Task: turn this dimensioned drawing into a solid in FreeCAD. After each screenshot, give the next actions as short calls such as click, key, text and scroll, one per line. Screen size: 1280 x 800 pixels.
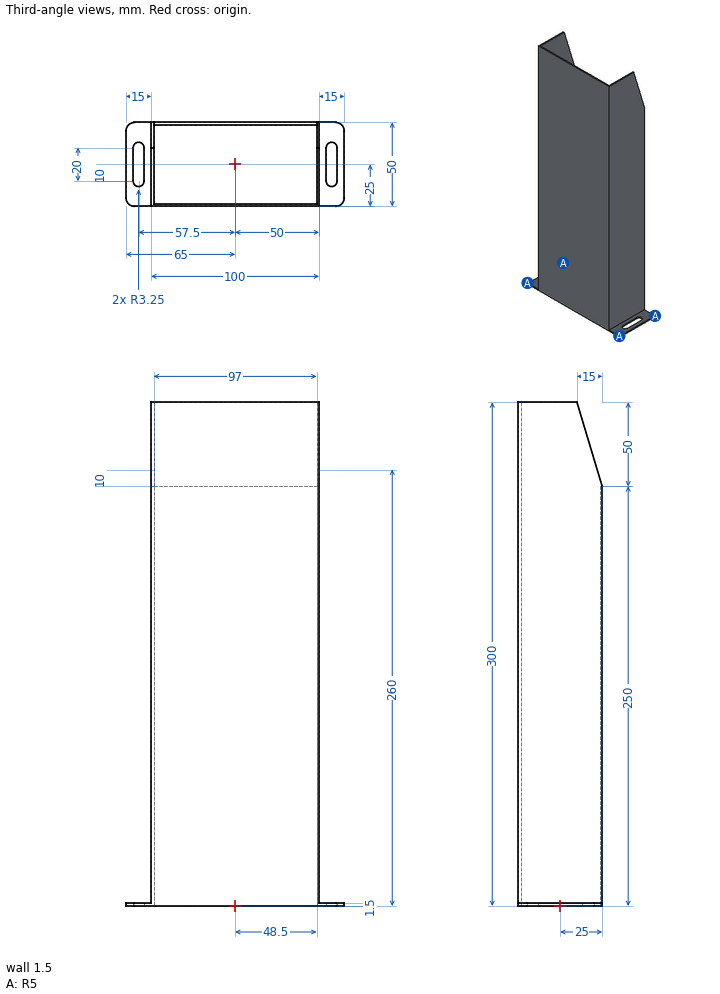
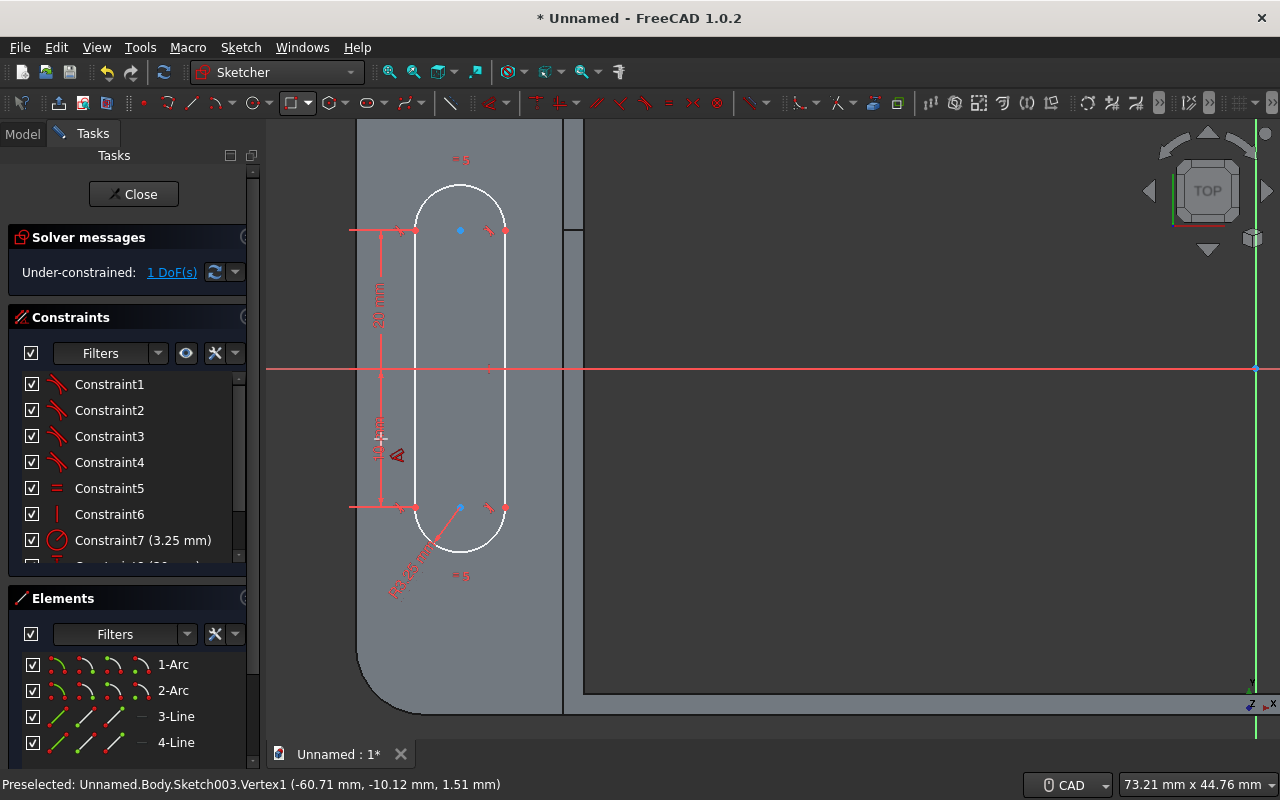
click(460, 507)
click(788, 541)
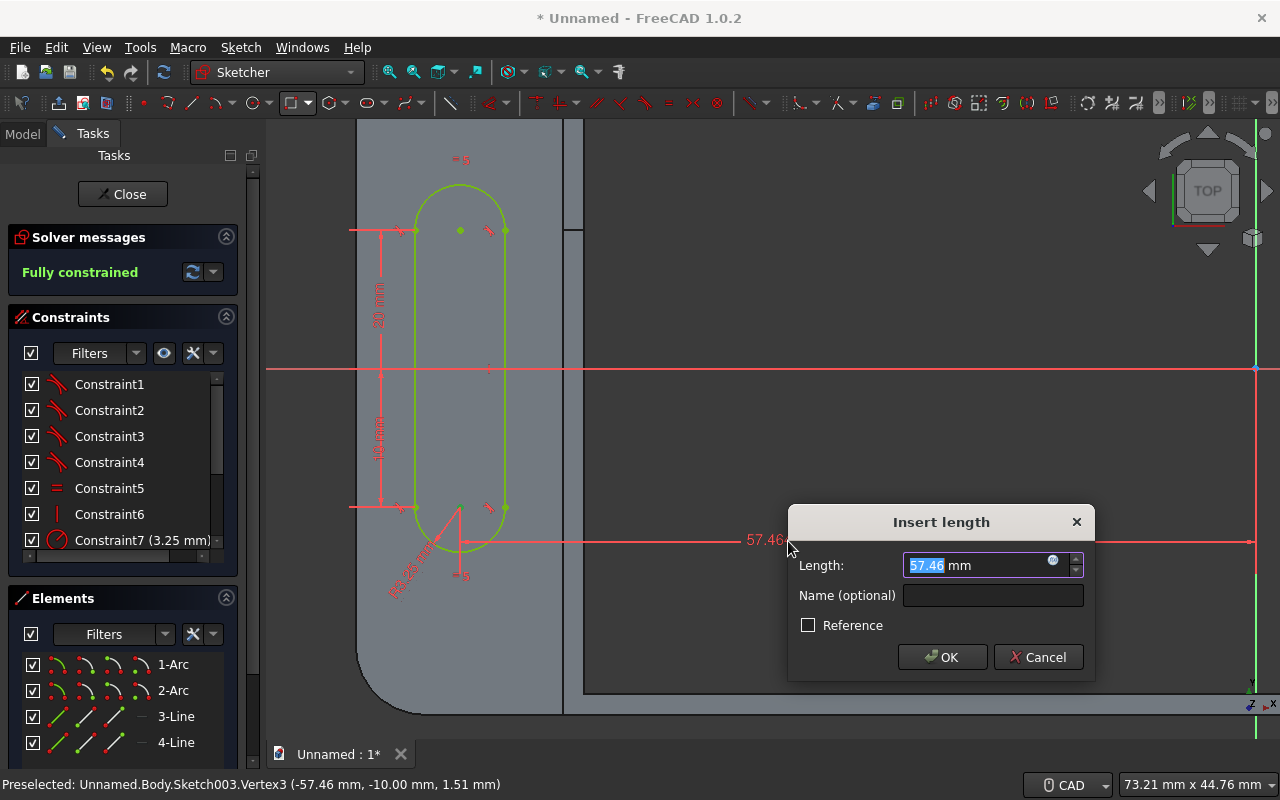
text(57.5)
key(Return)
key(Escape)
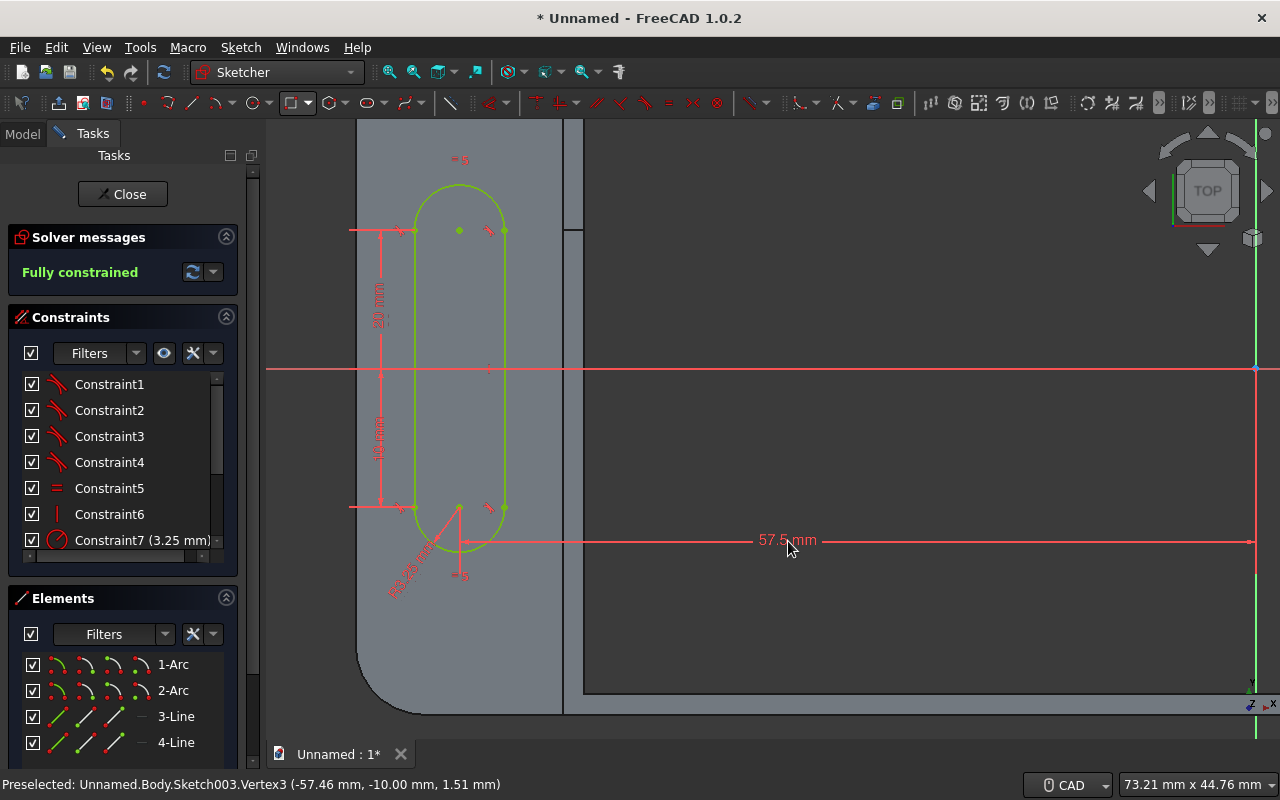
click(123, 194)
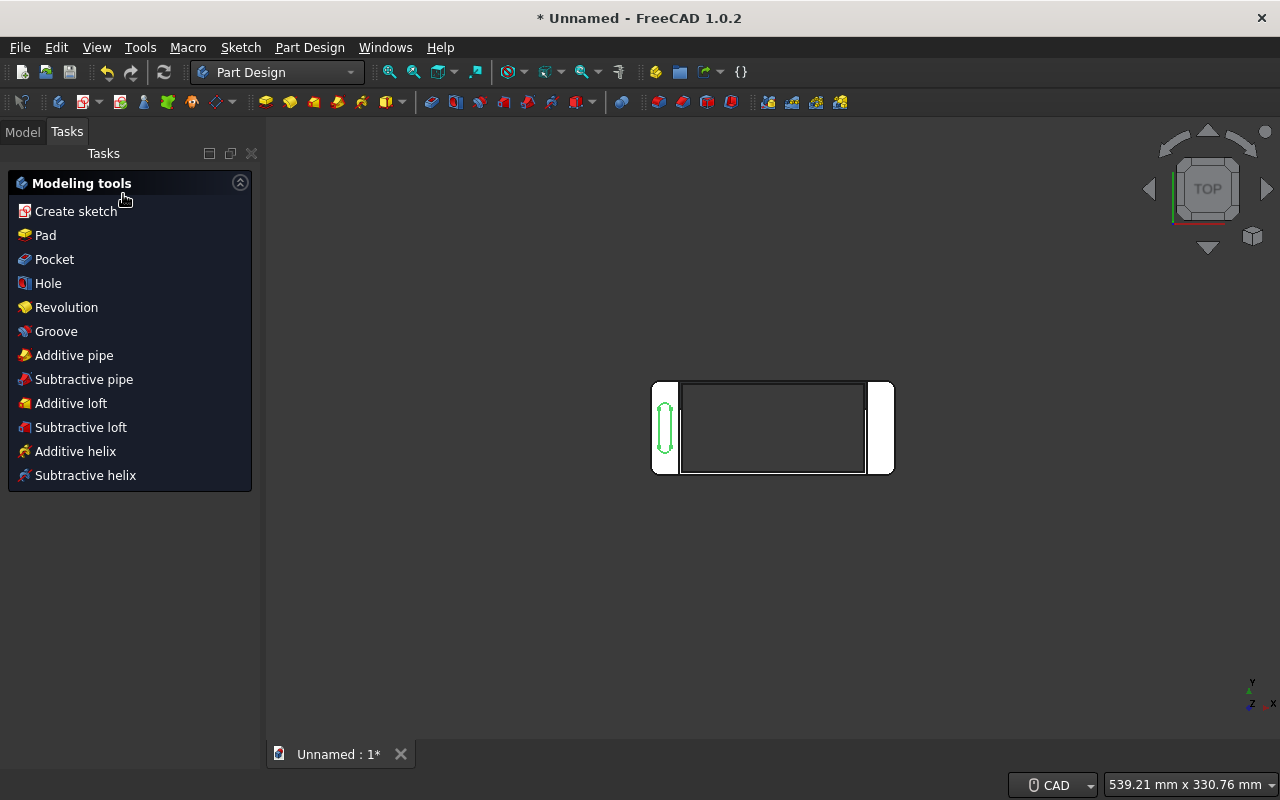
click(432, 102)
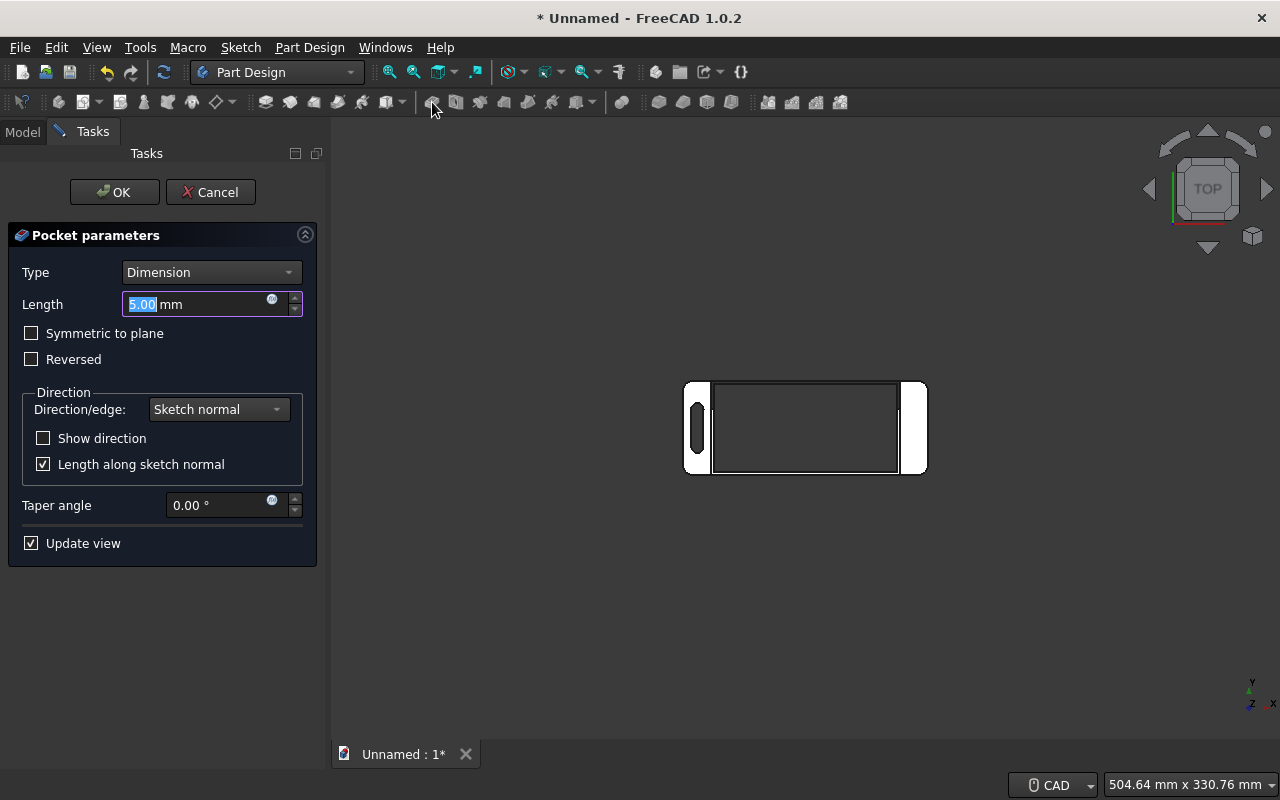
click(212, 272)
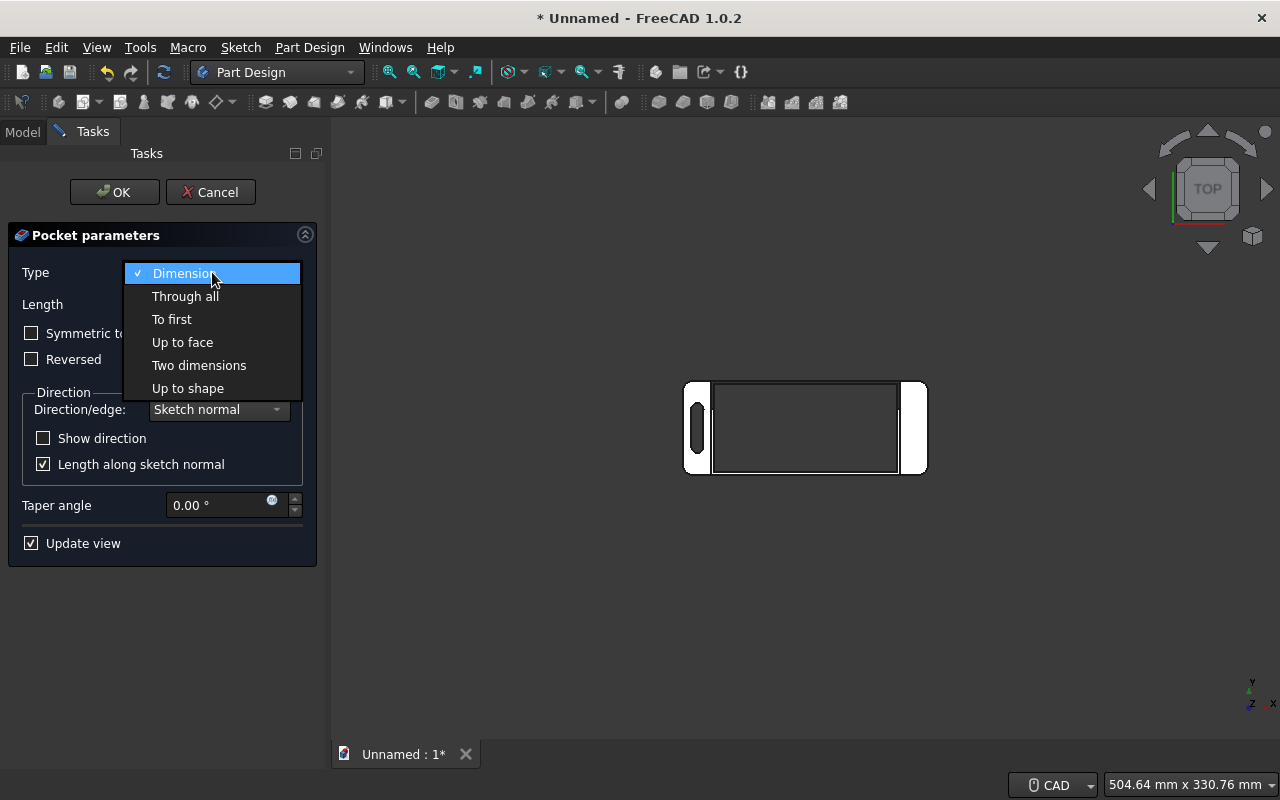
click(212, 296)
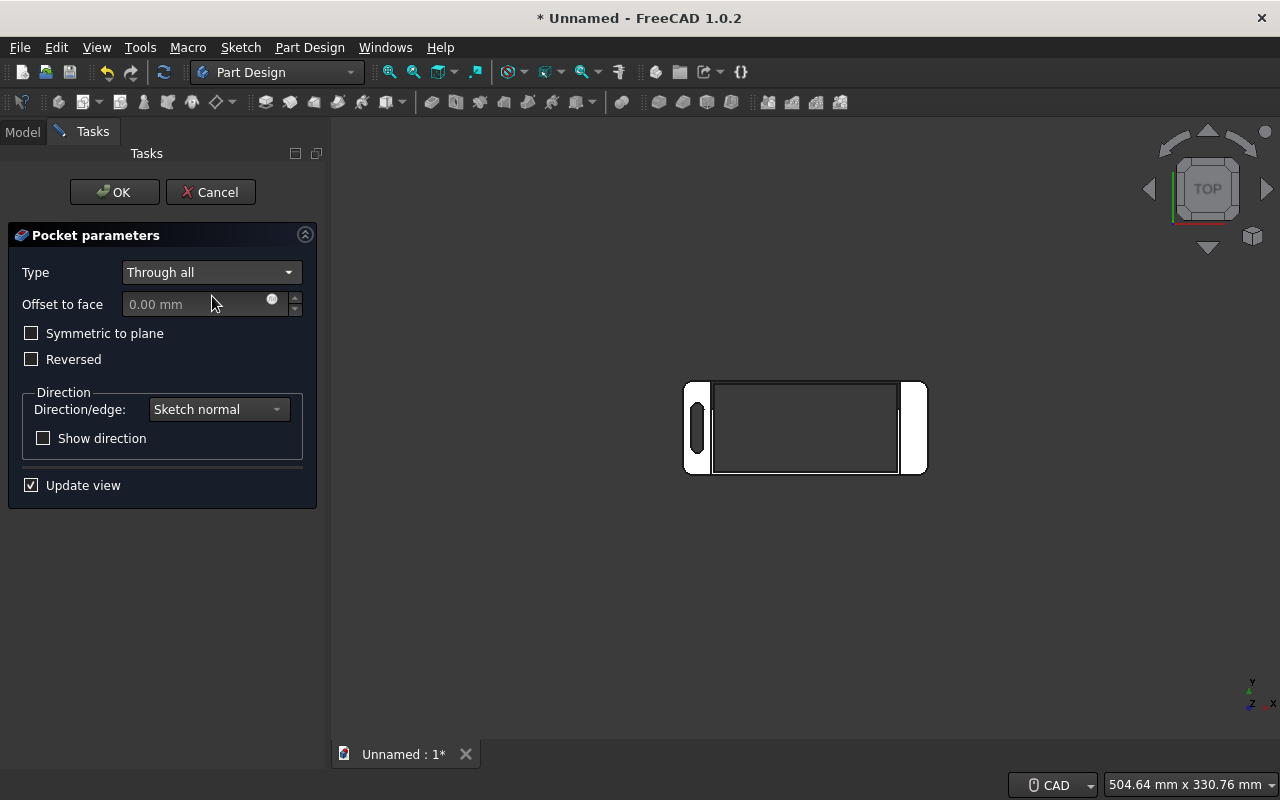
click(115, 192)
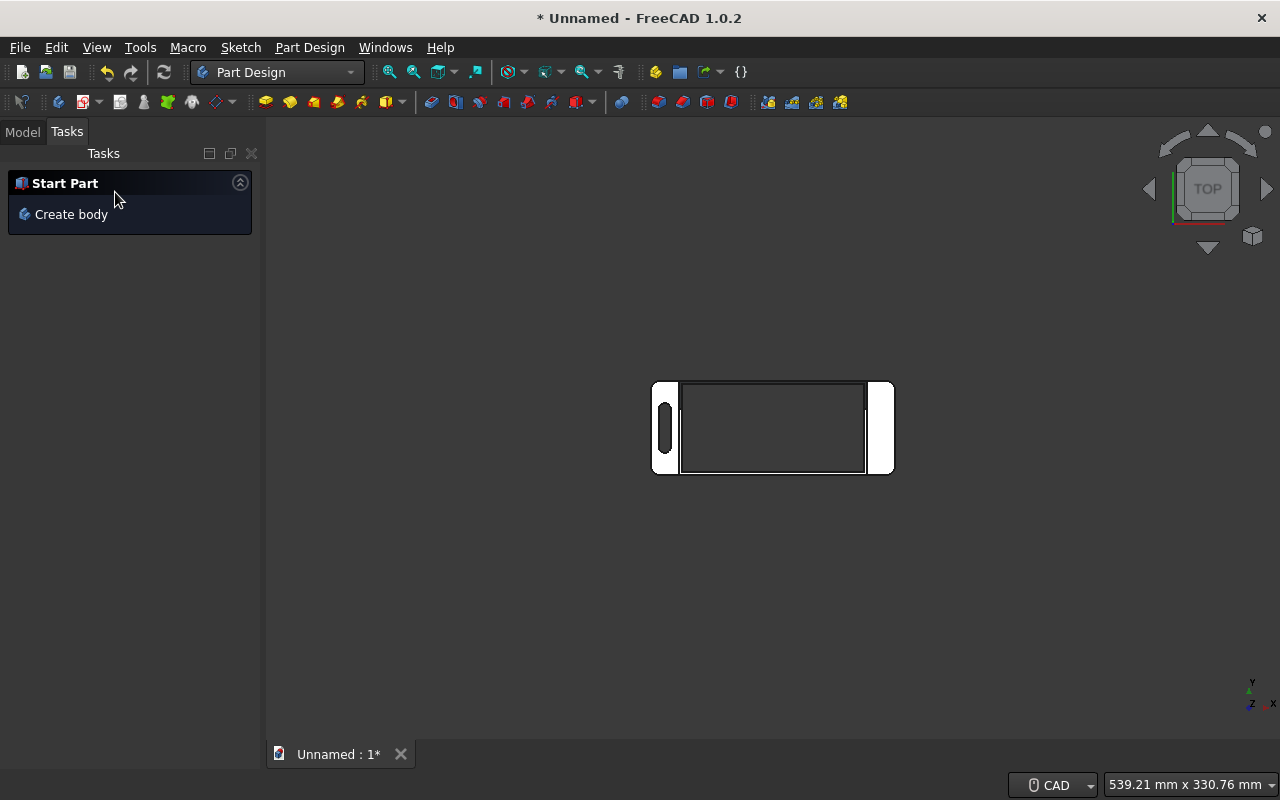
click(390, 72)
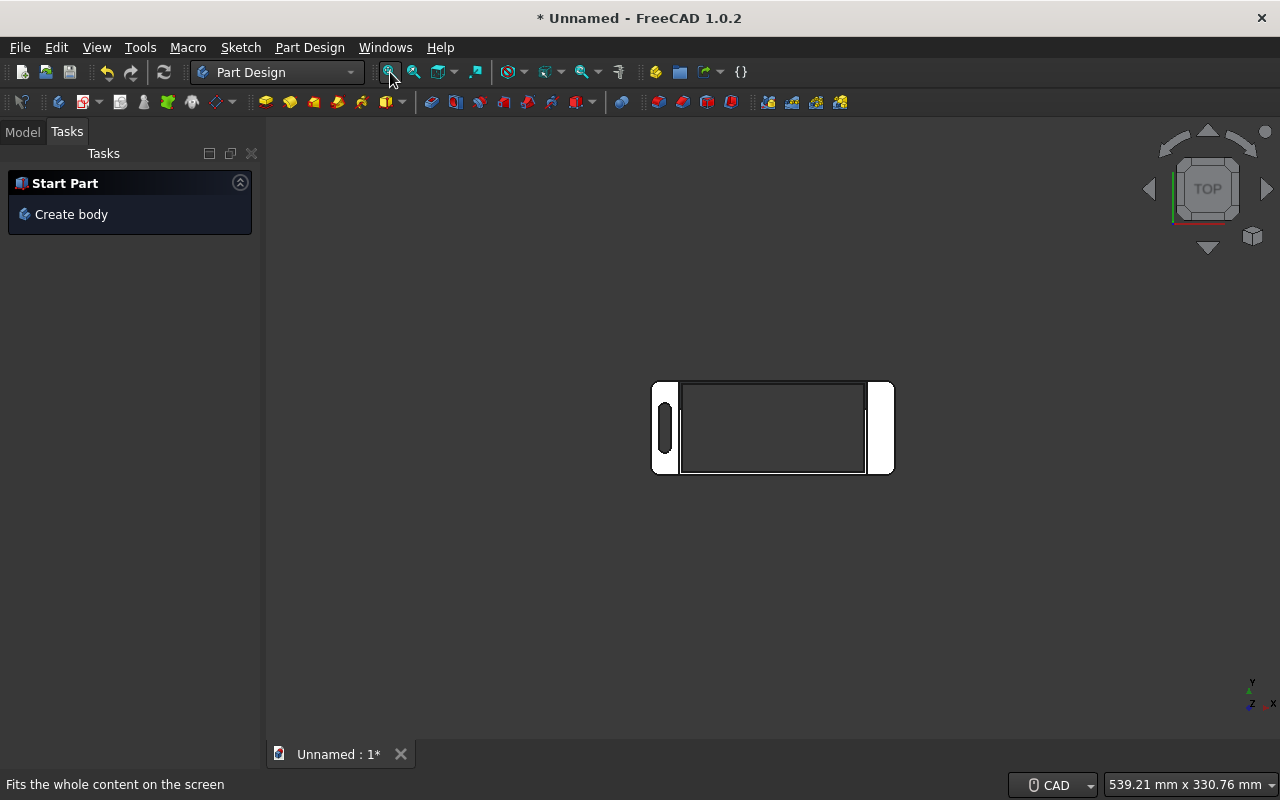
click(23, 131)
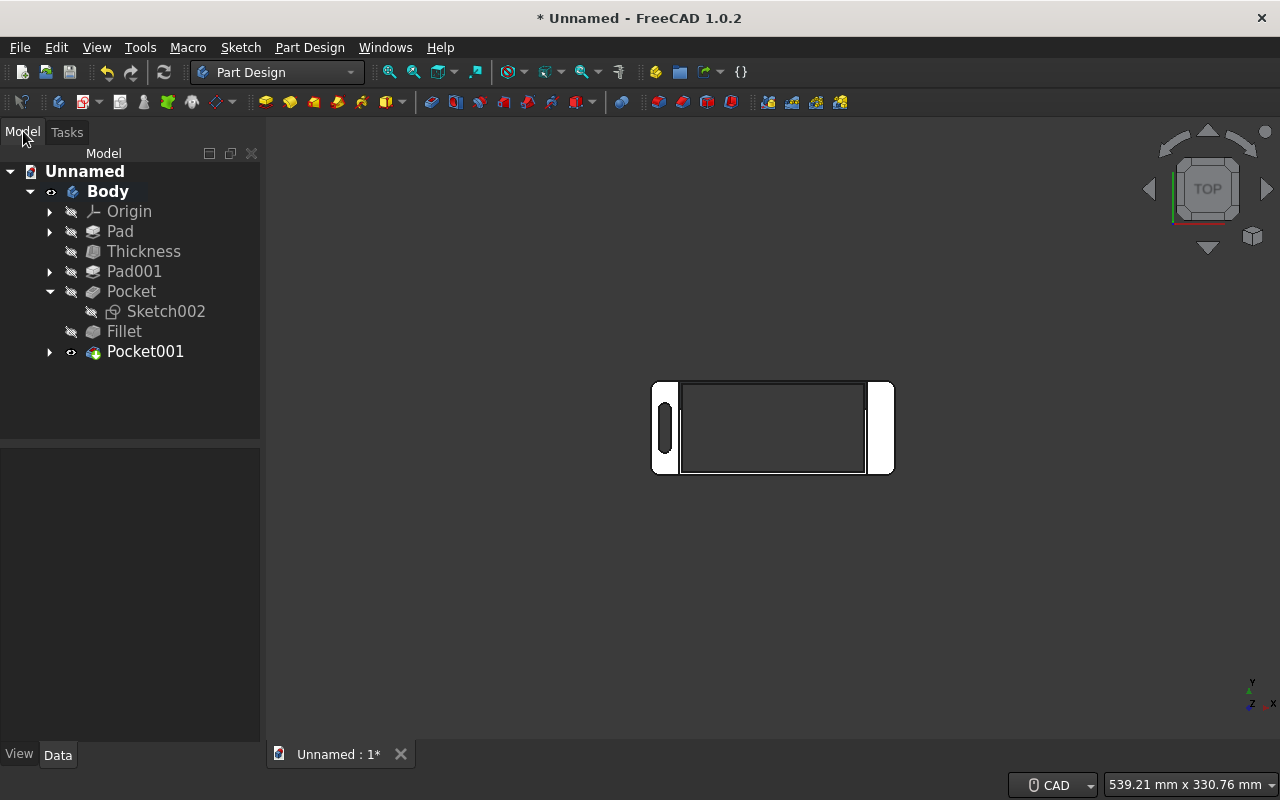
click(116, 352)